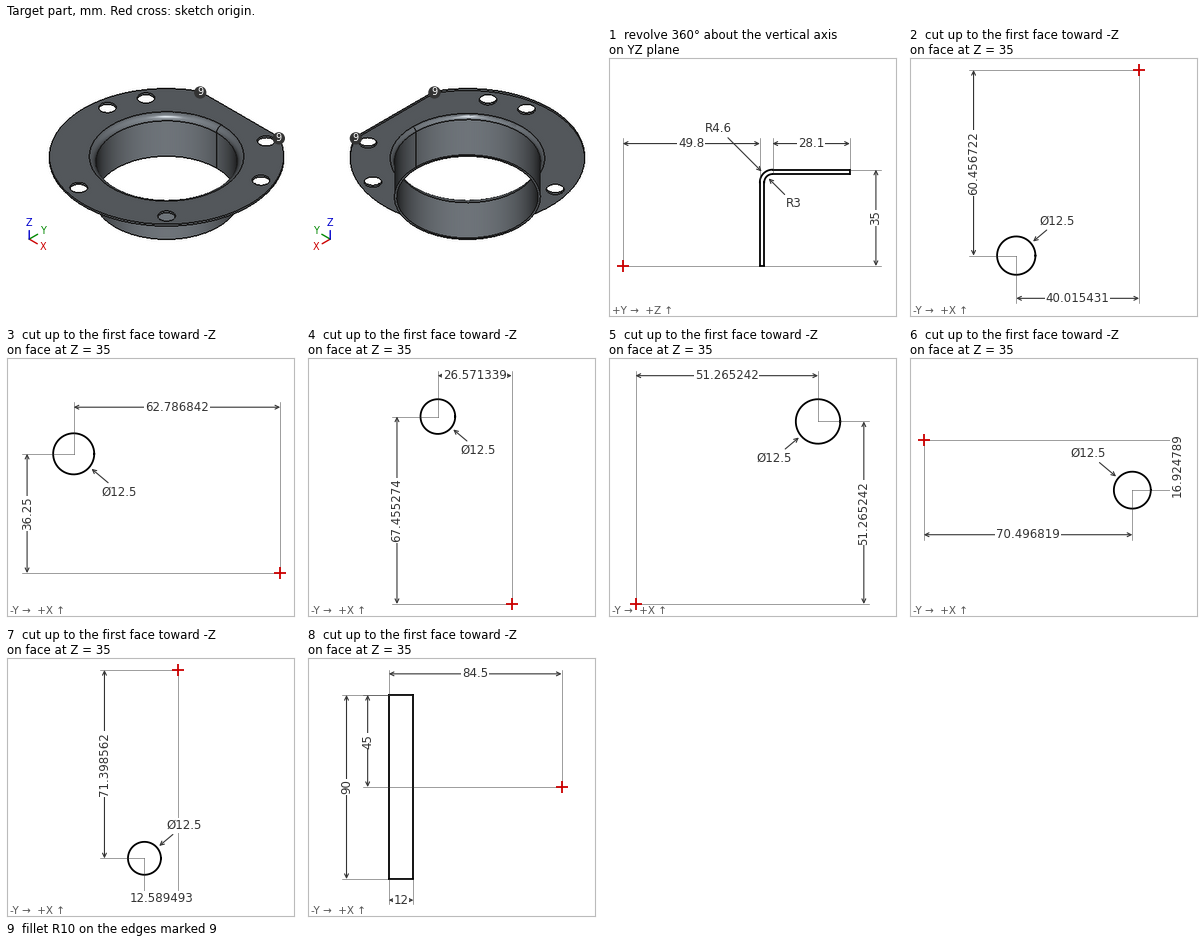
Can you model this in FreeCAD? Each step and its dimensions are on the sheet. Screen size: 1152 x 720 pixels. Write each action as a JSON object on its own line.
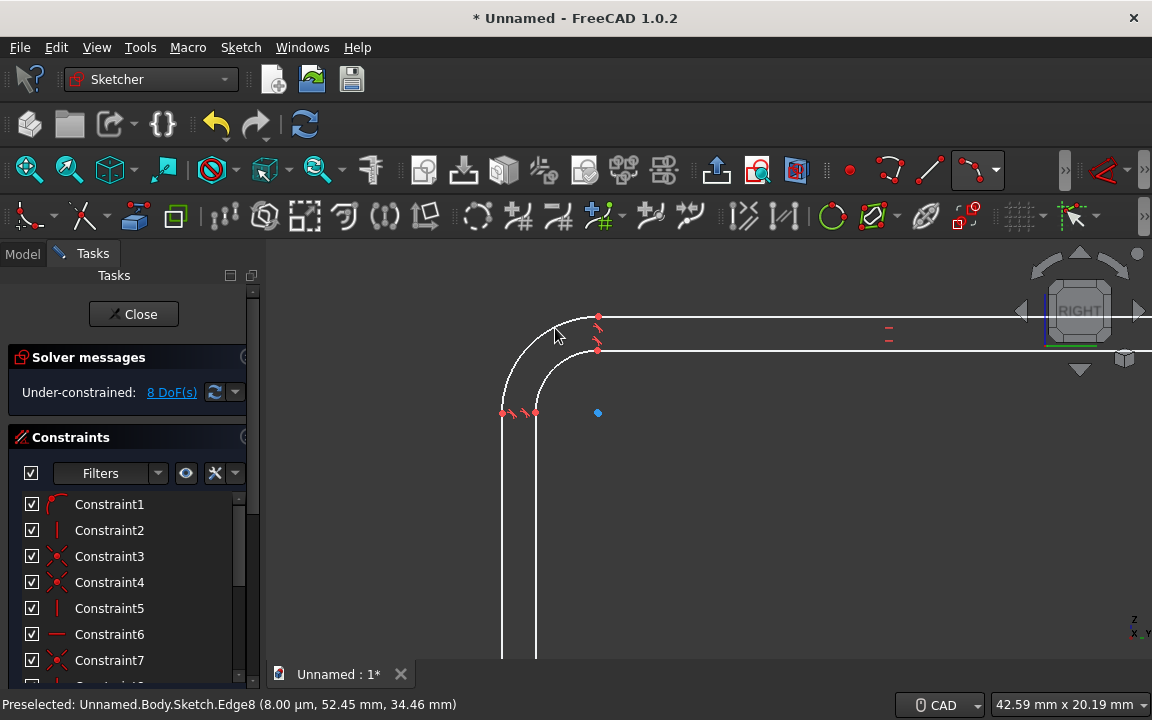
{"action": "scroll", "coordinate": [777, 350], "scroll_direction": "down", "scroll_amount": 6}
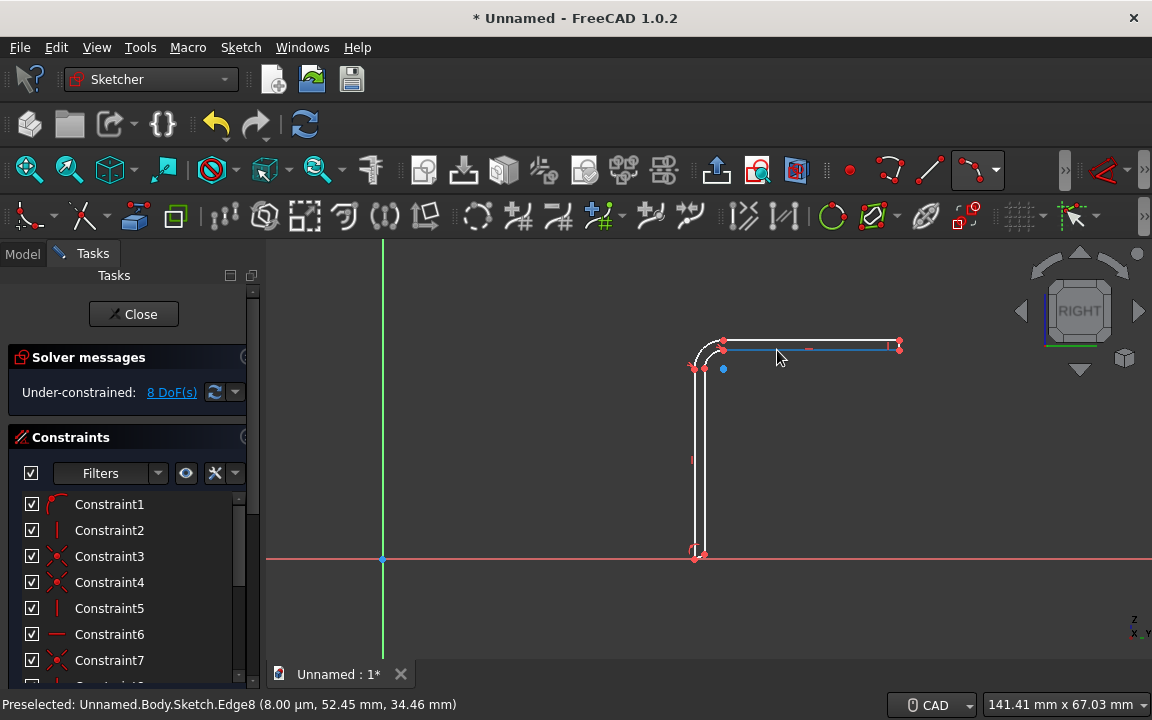
{"action": "scroll", "coordinate": [702, 556], "scroll_direction": "up", "scroll_amount": 8}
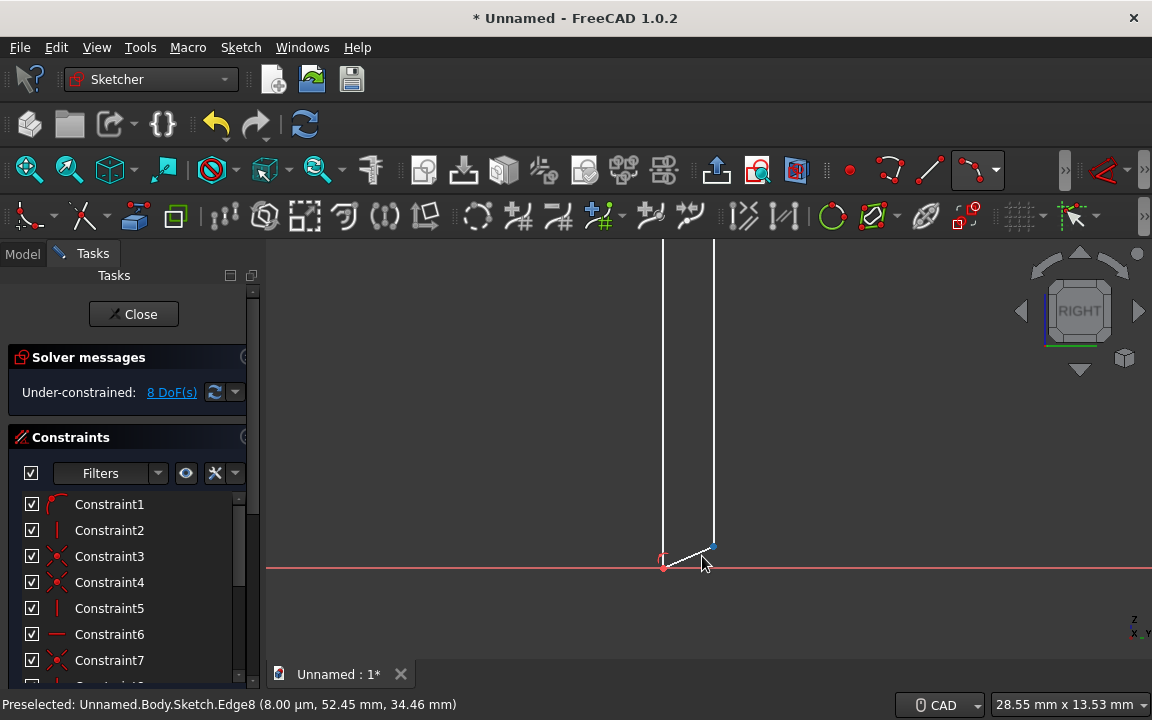
{"action": "left_click", "coordinate": [699, 553]}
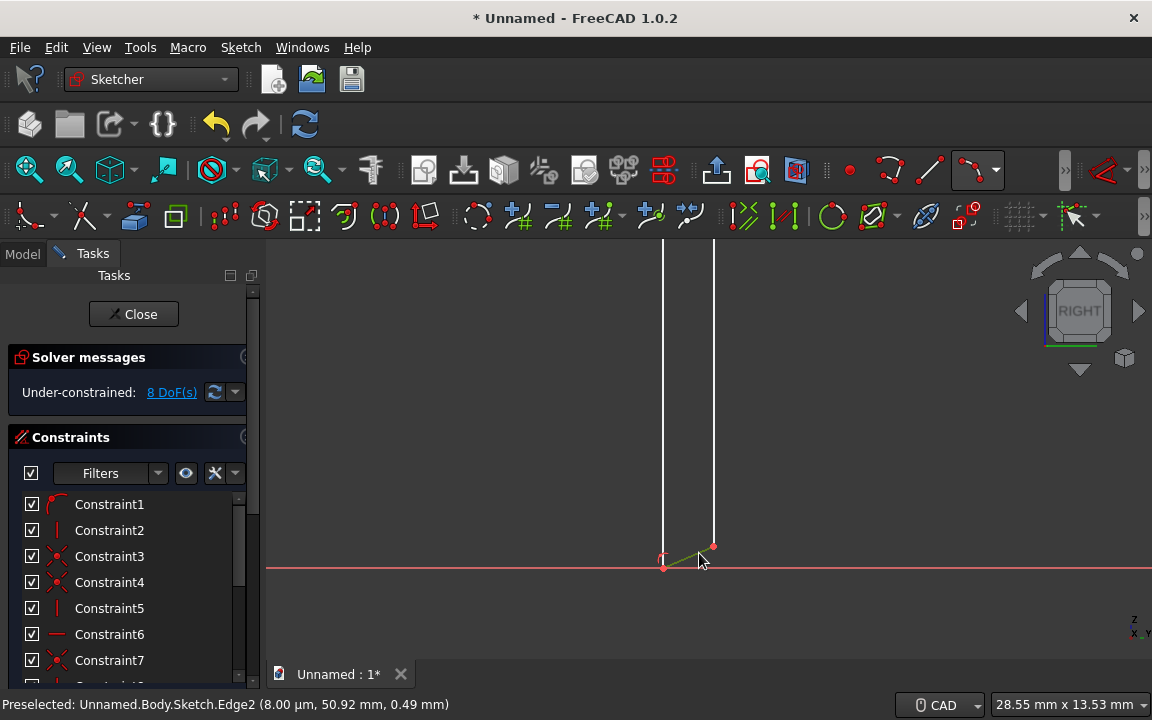
{"action": "key", "text": "h"}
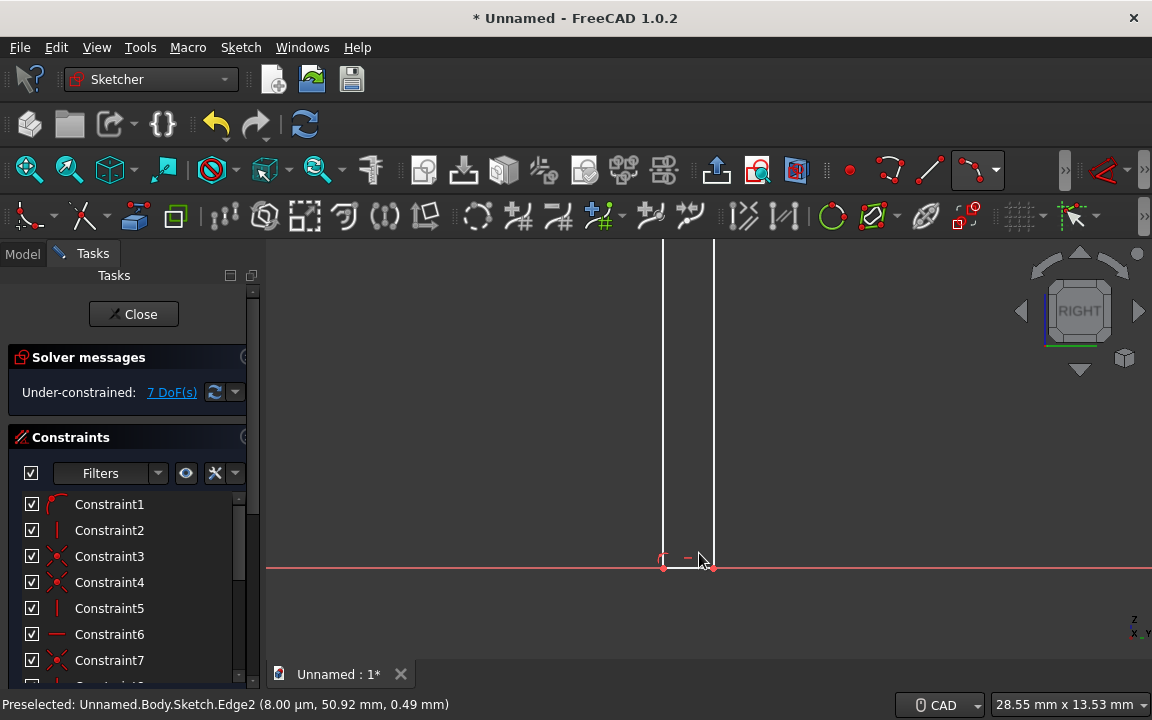
{"action": "scroll", "coordinate": [702, 556], "scroll_direction": "down", "scroll_amount": 8}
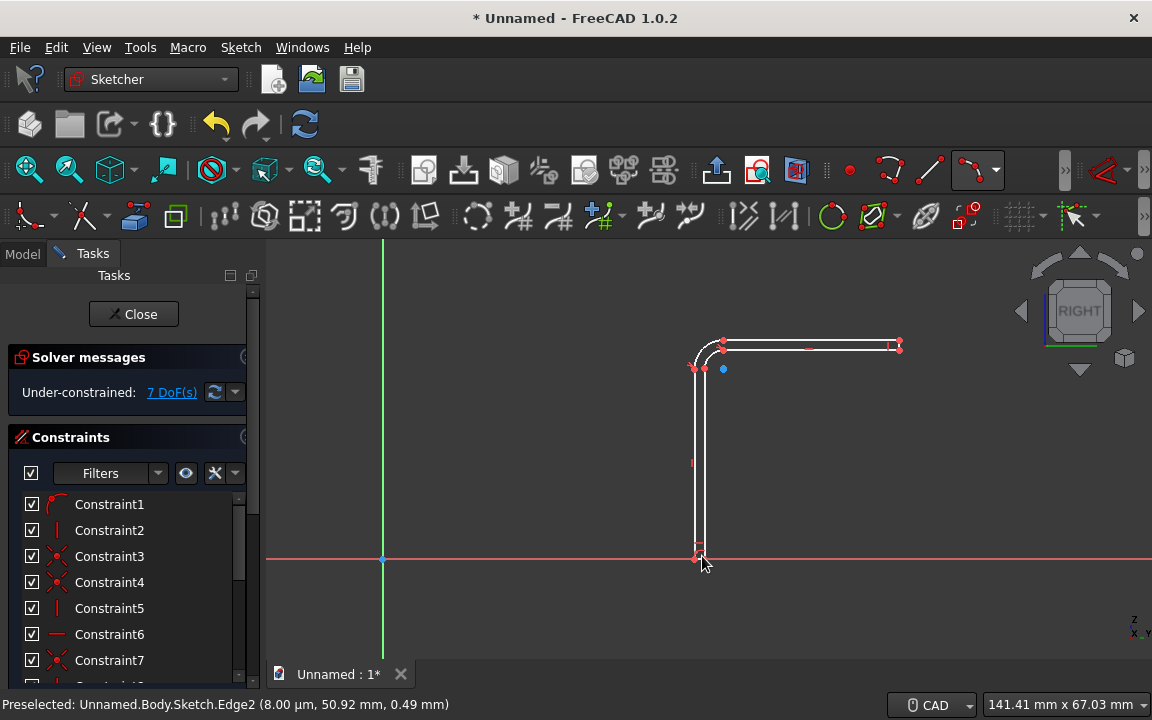
{"action": "scroll", "coordinate": [715, 352], "scroll_direction": "up", "scroll_amount": 3}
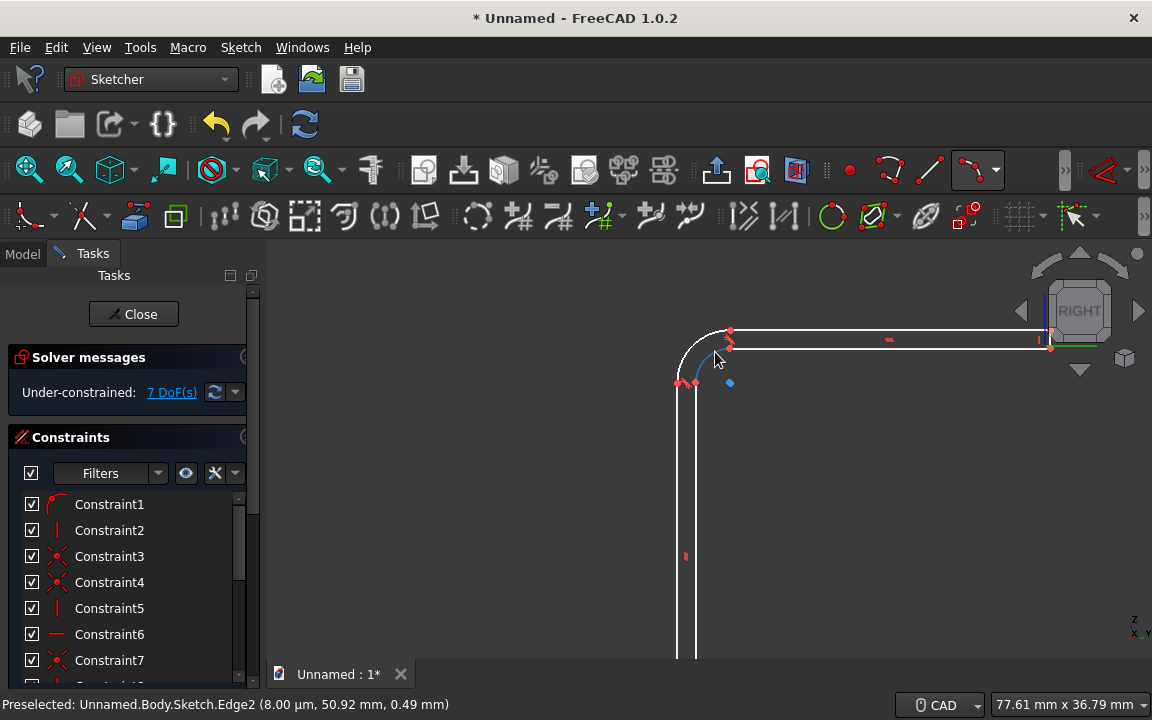
{"action": "left_click", "coordinate": [714, 353]}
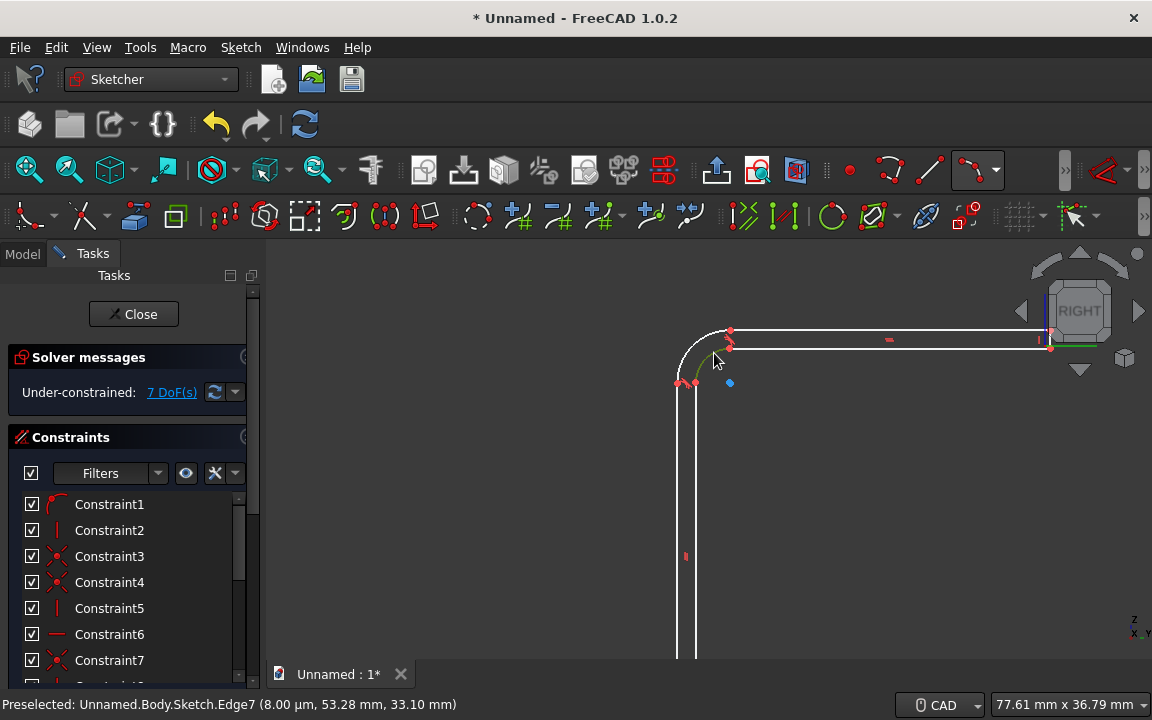
{"action": "left_click", "coordinate": [706, 336]}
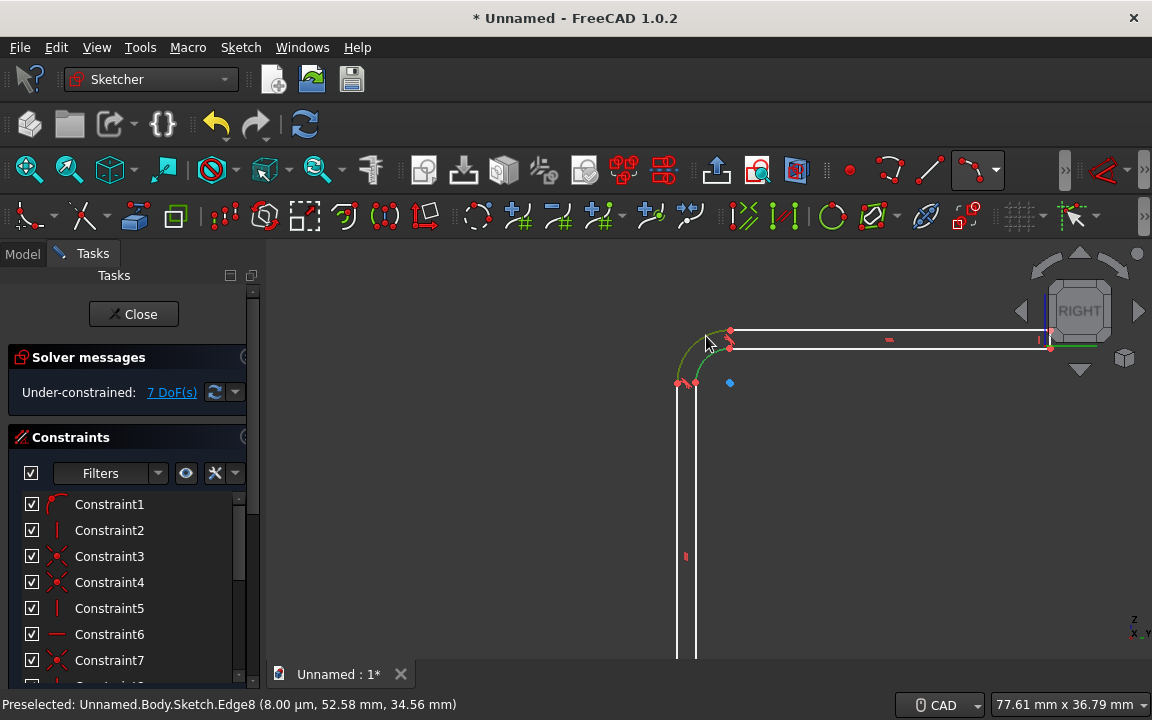
{"action": "key", "text": "c"}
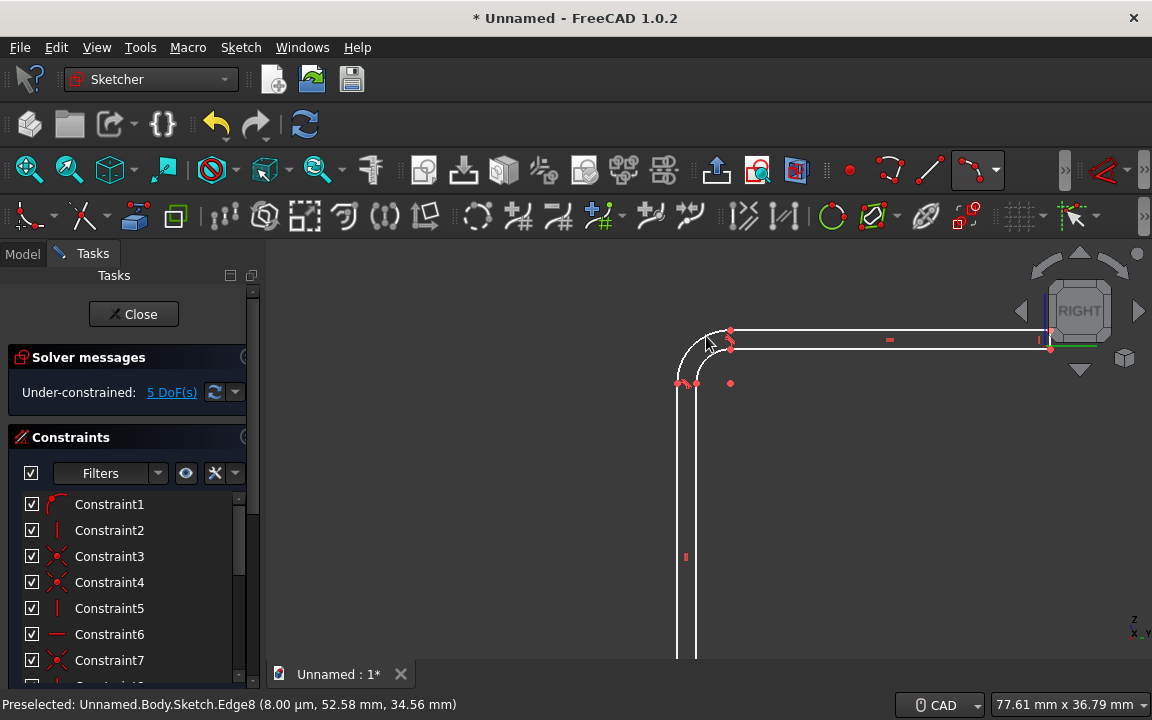
{"action": "left_click", "coordinate": [715, 353]}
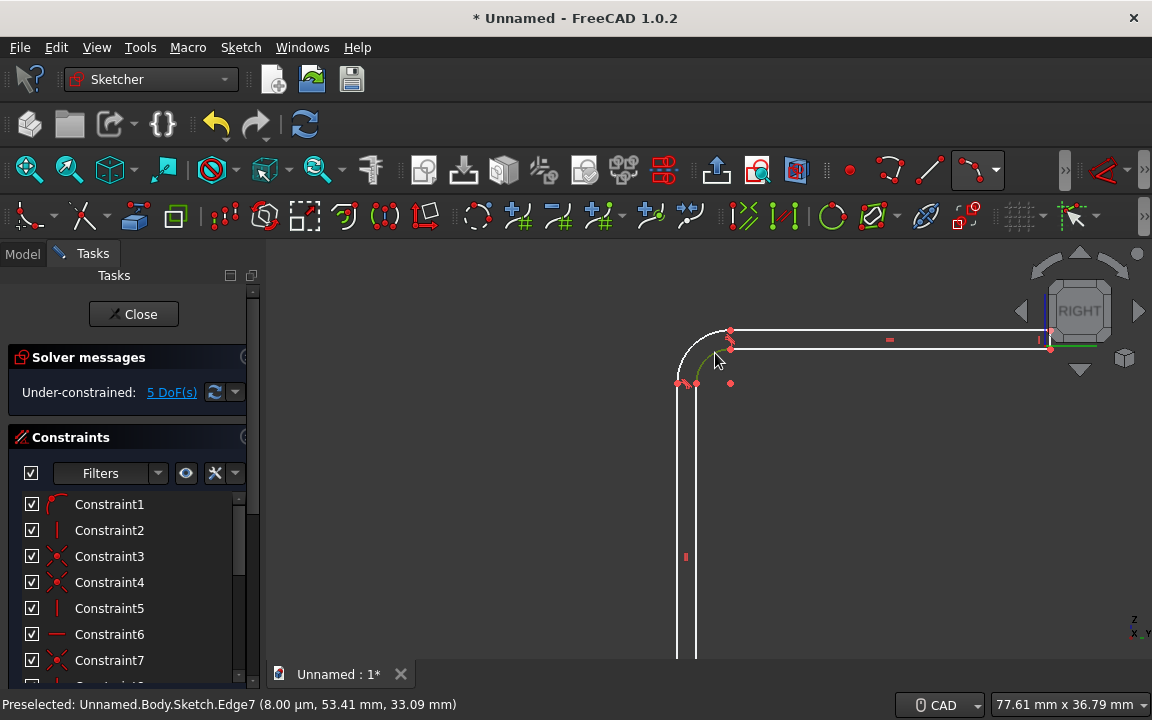
{"action": "key", "text": "k r"}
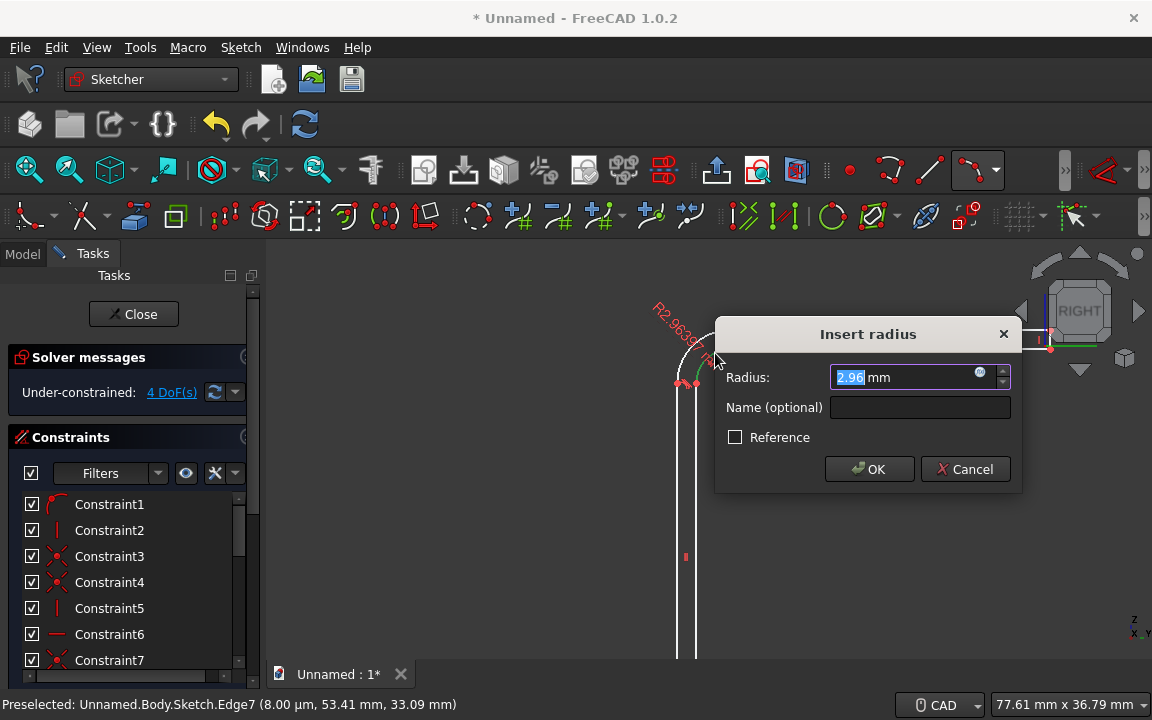
{"action": "type", "text": "3"}
{"action": "key", "text": "Return"}